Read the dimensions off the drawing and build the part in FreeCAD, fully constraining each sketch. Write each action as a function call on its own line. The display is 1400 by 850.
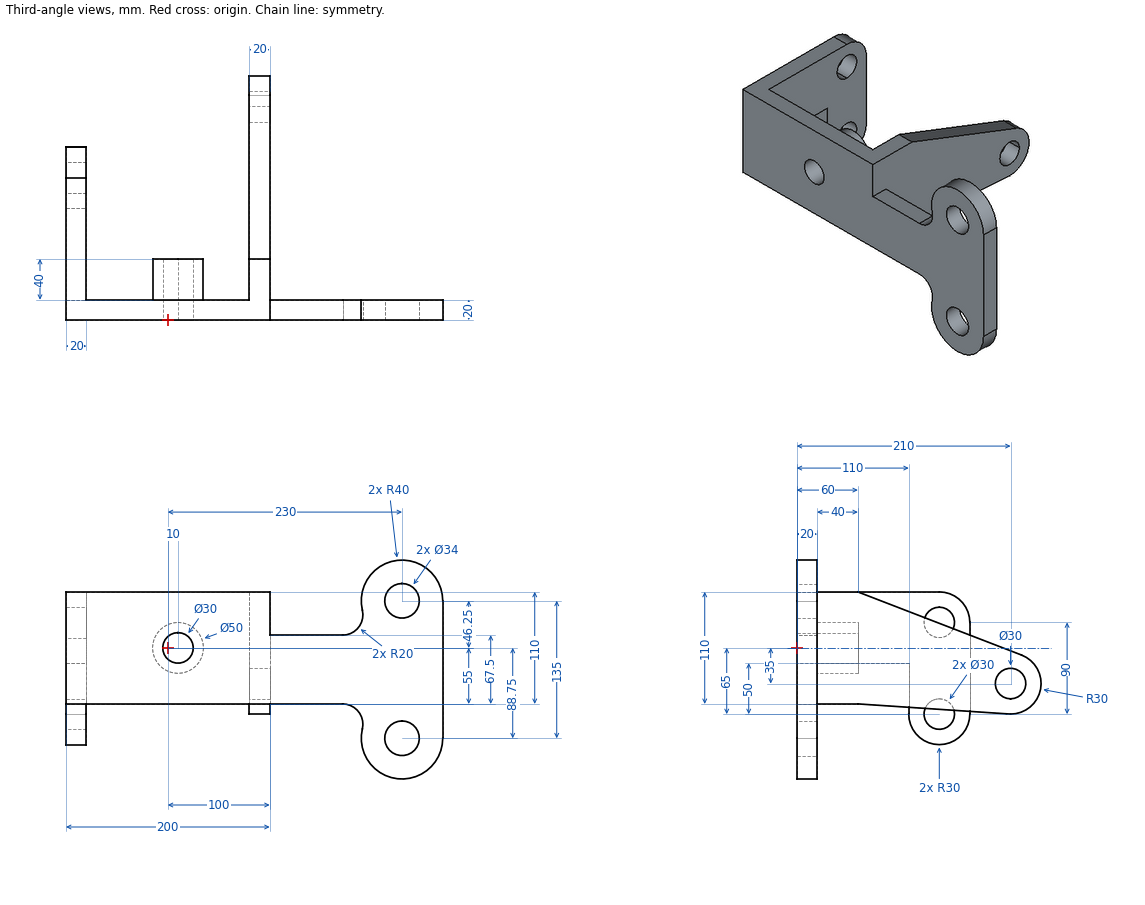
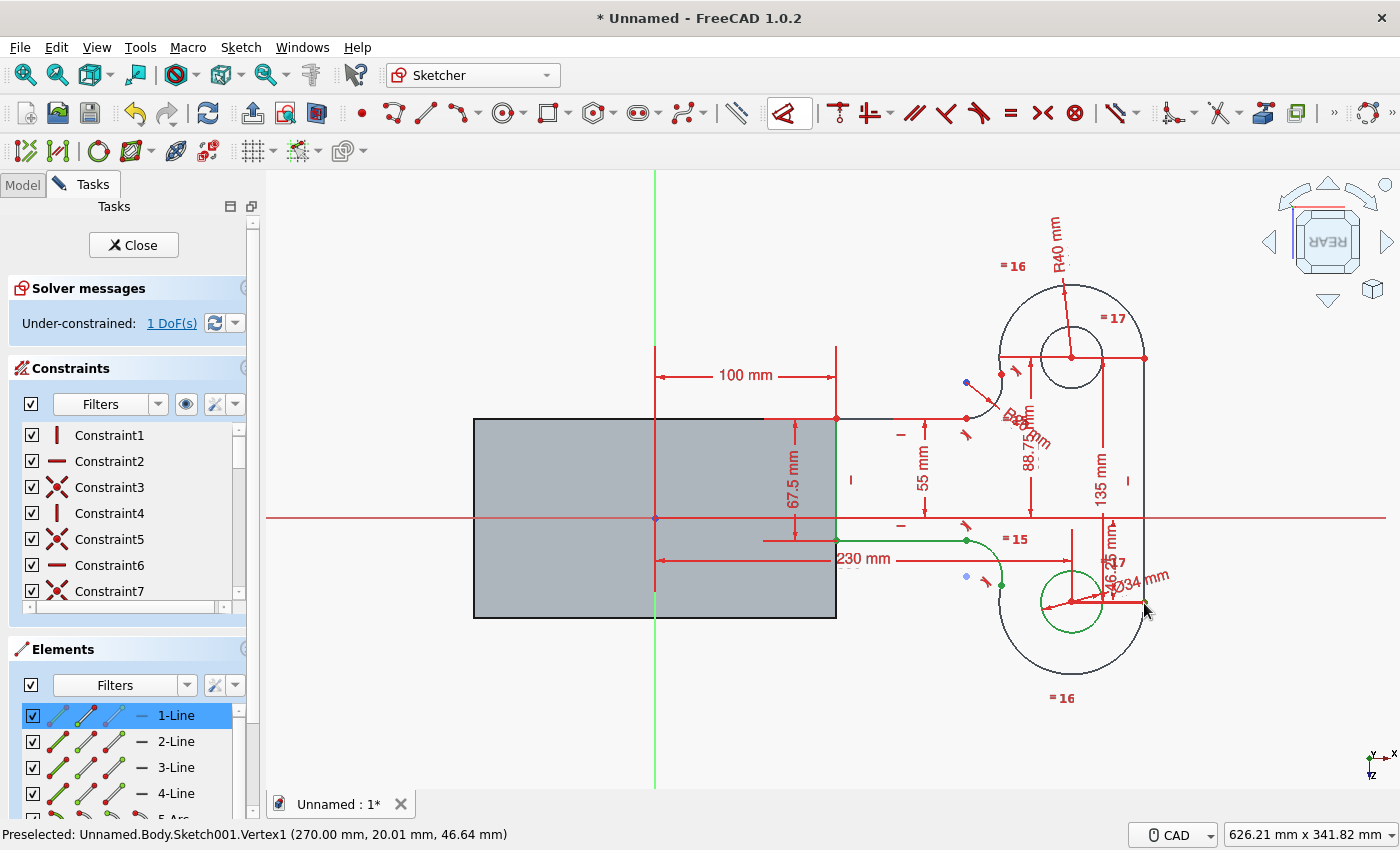
key(i)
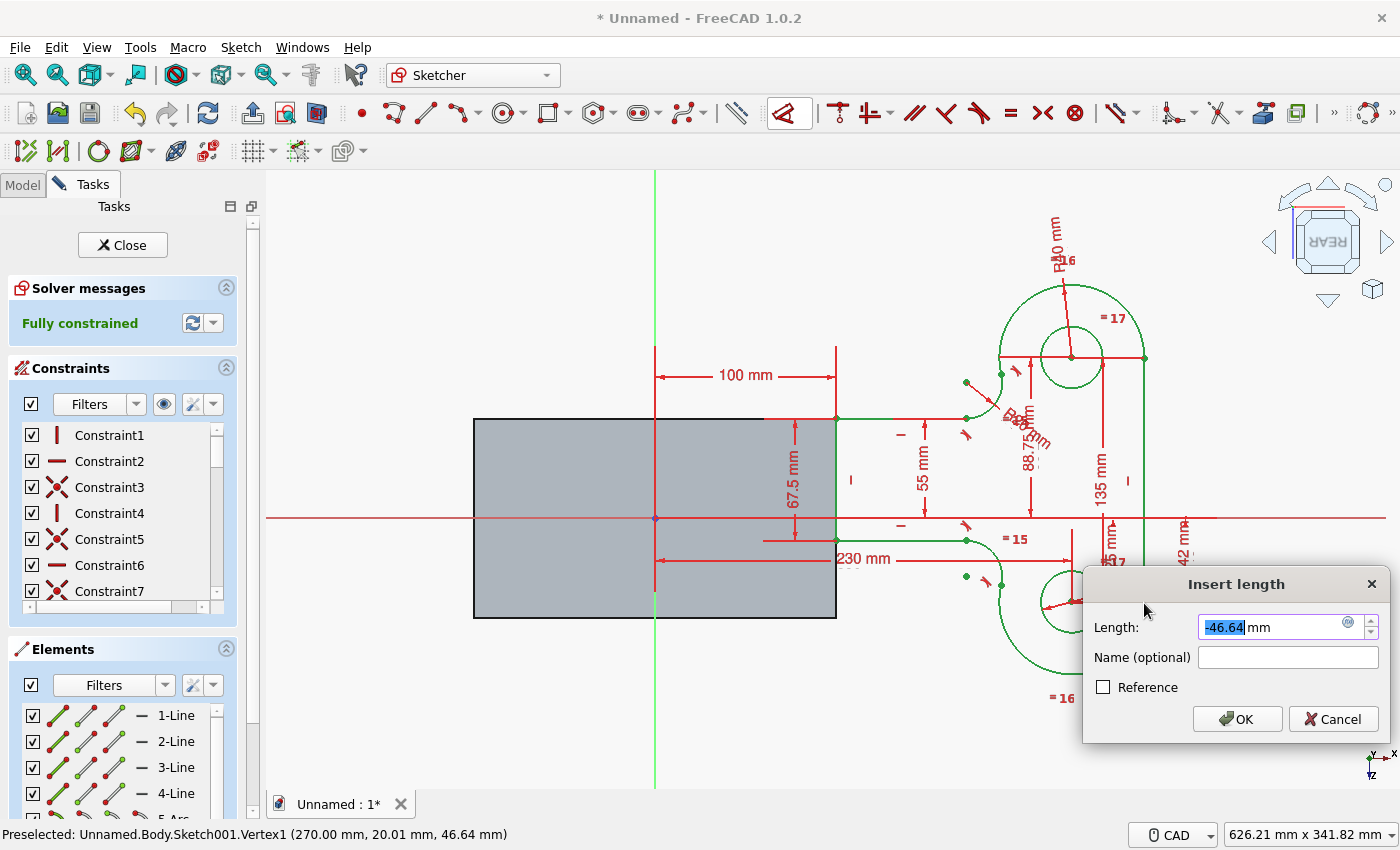
text(-46.25)
key(Return)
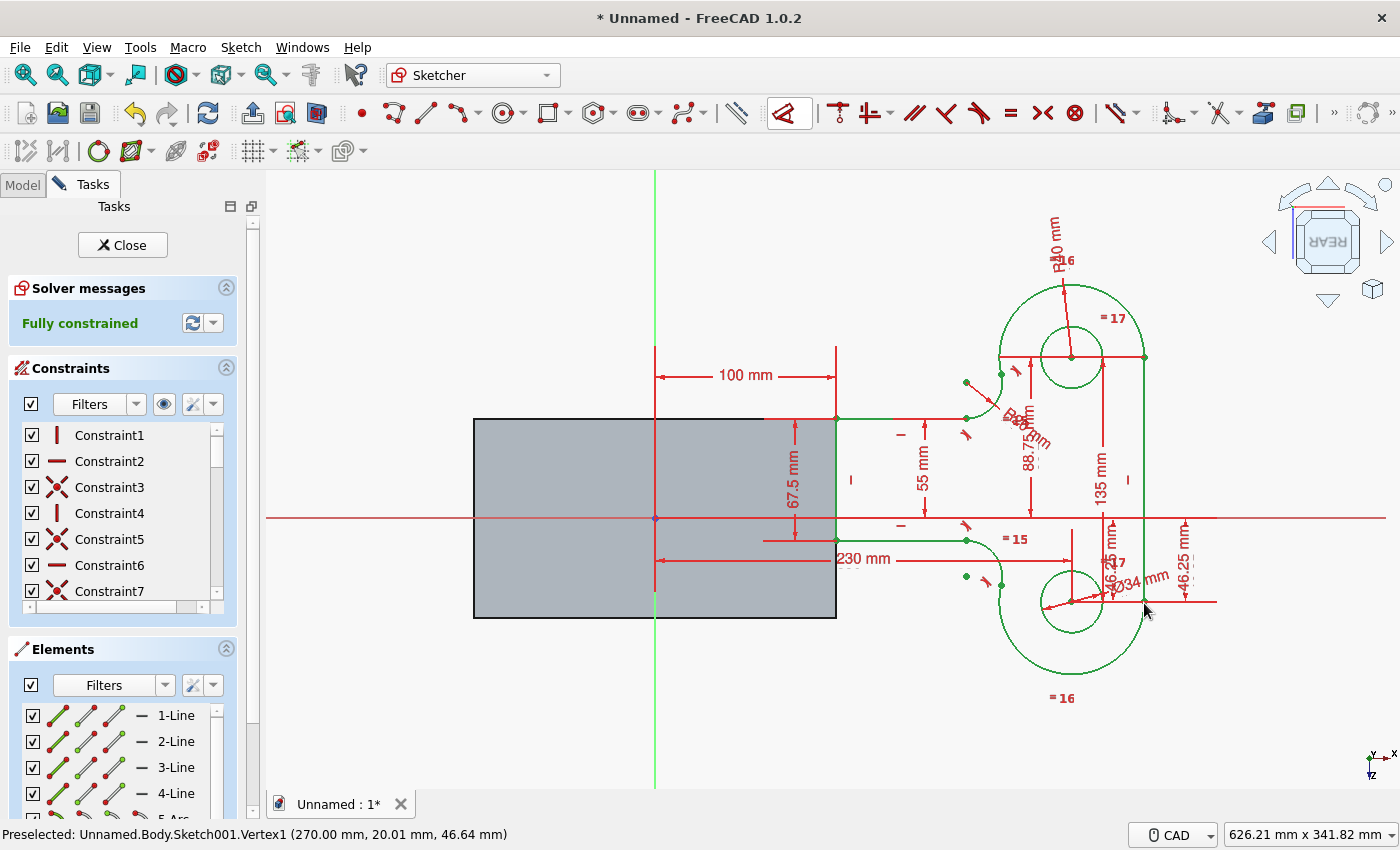
click(123, 245)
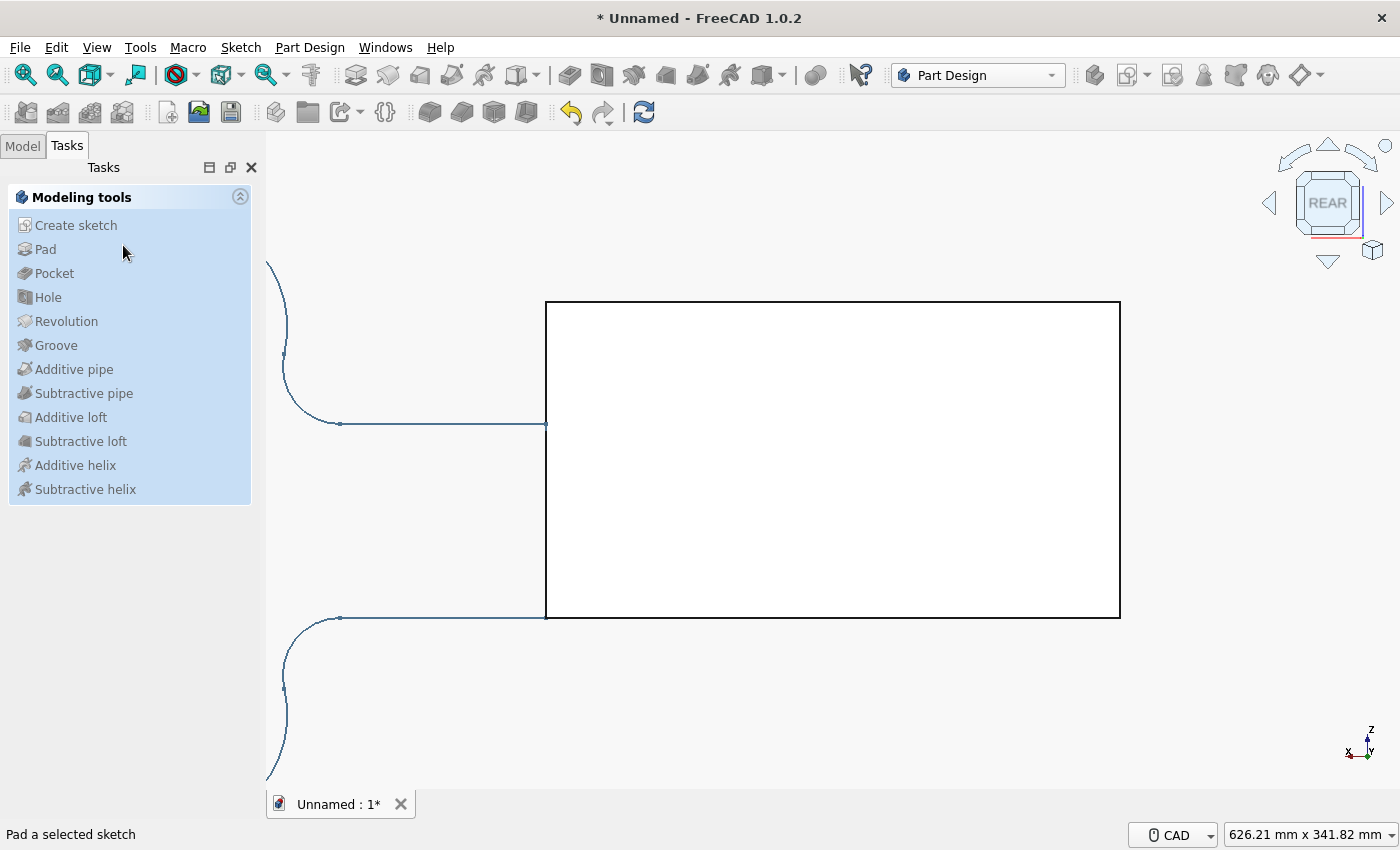
click(356, 76)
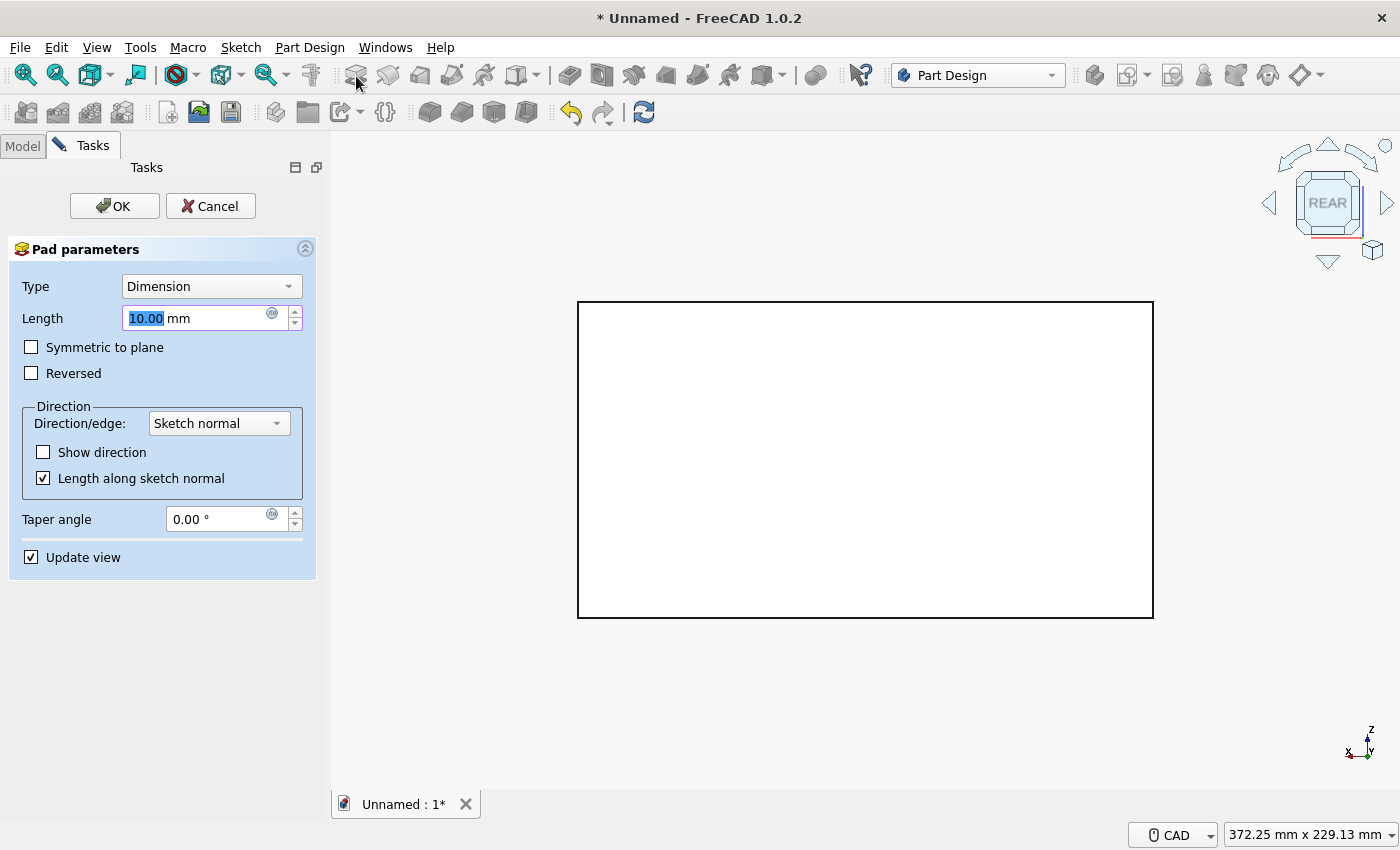
text(20)
key(Tab)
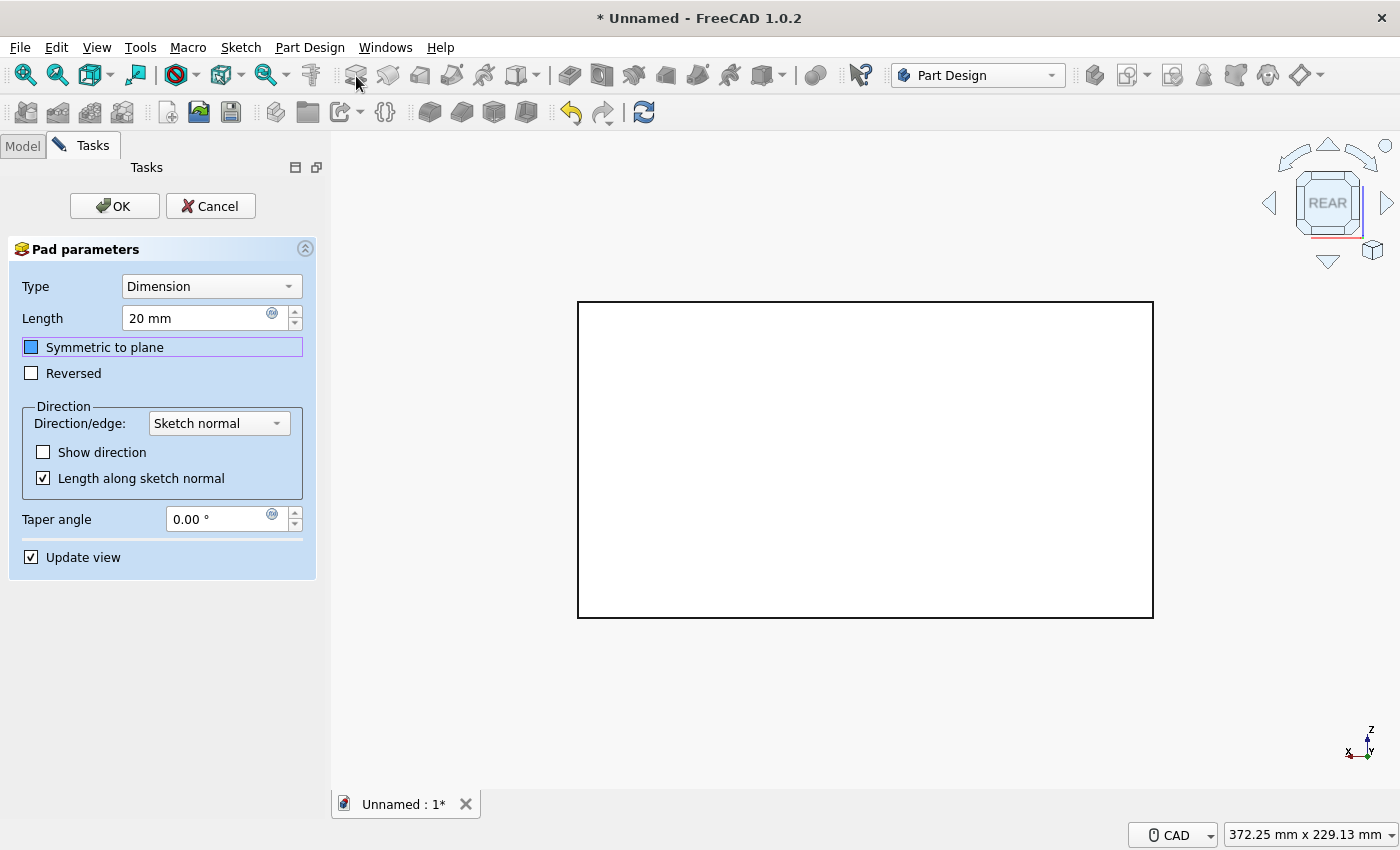
click(30, 373)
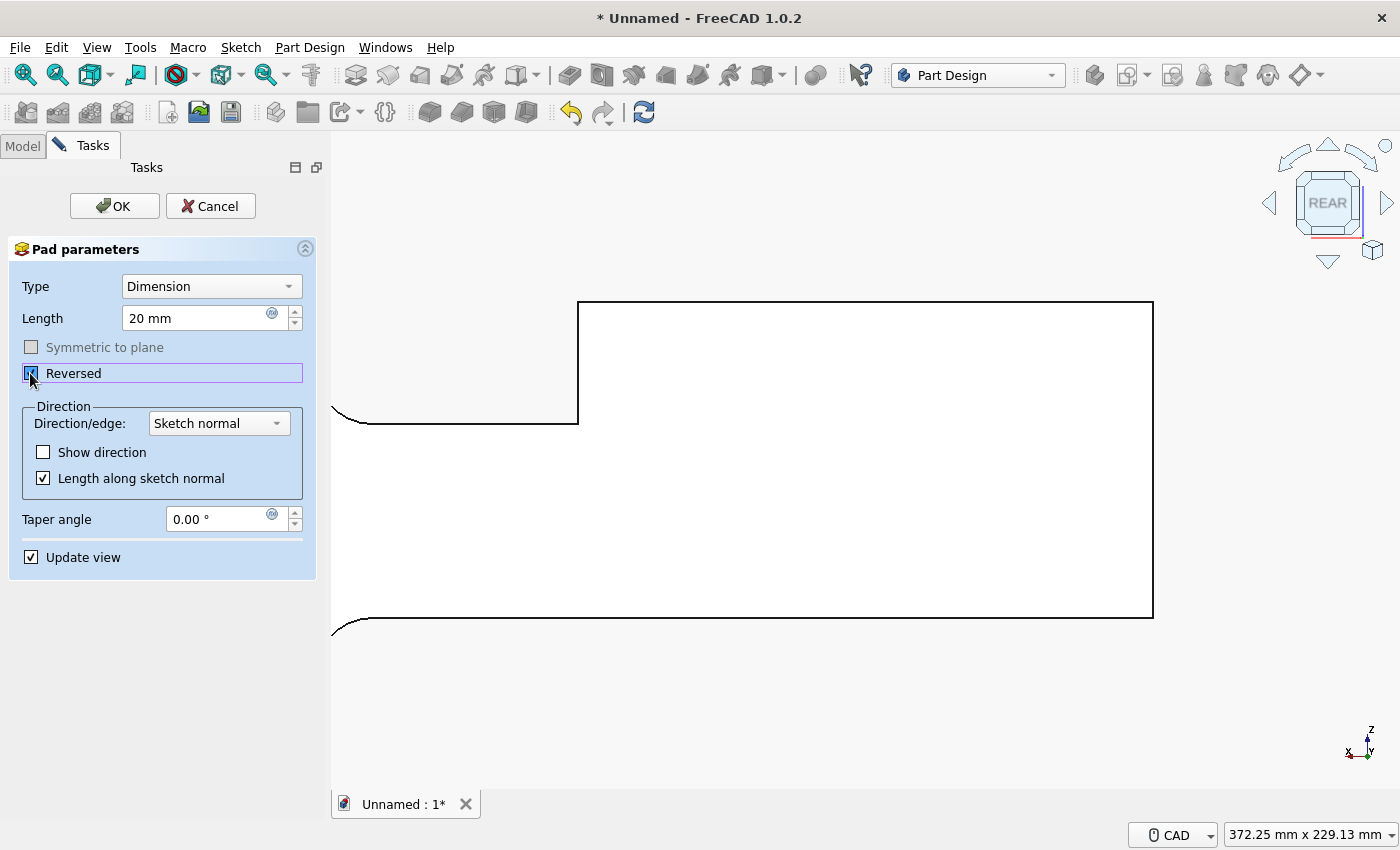
click(115, 206)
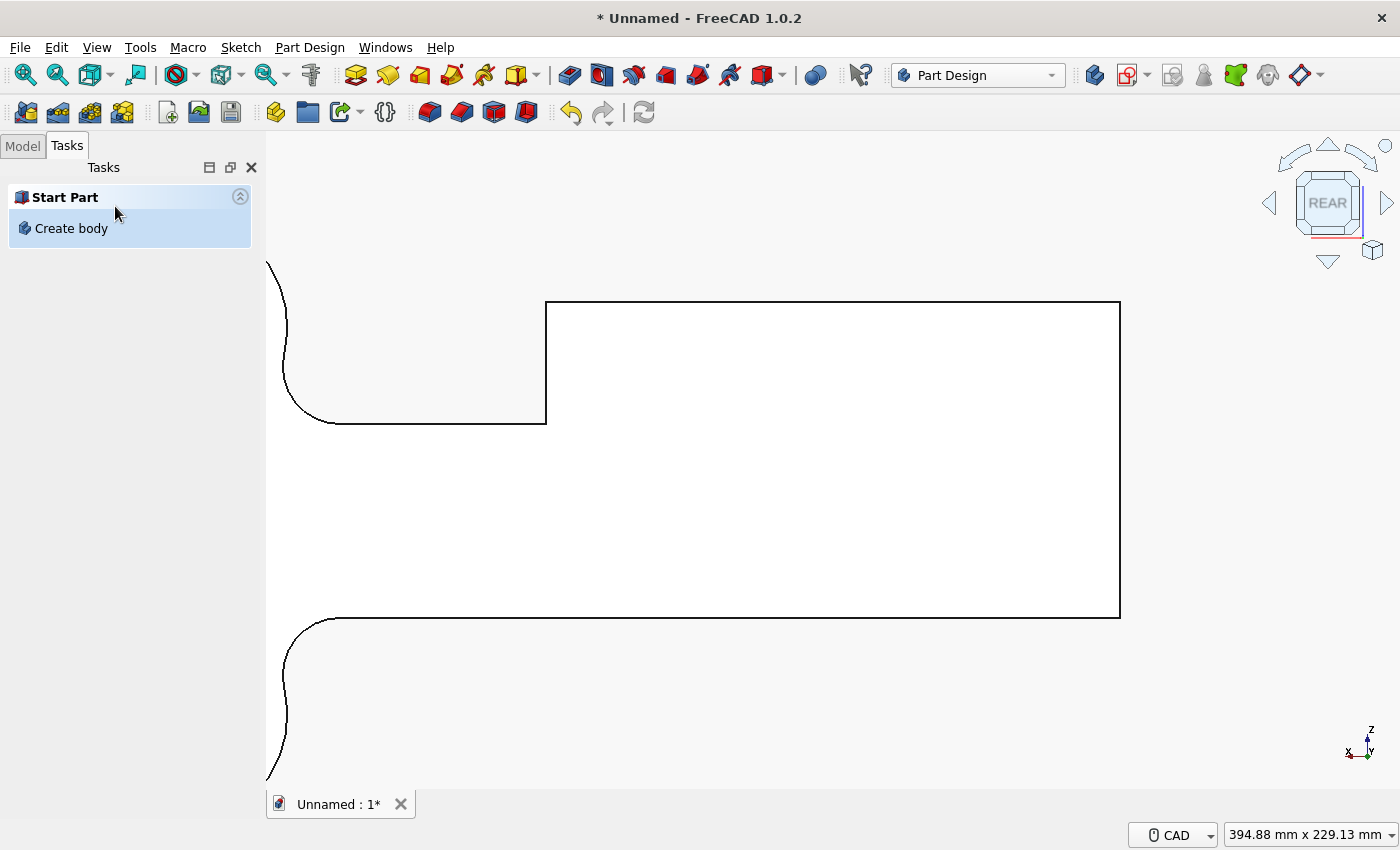
click(26, 76)